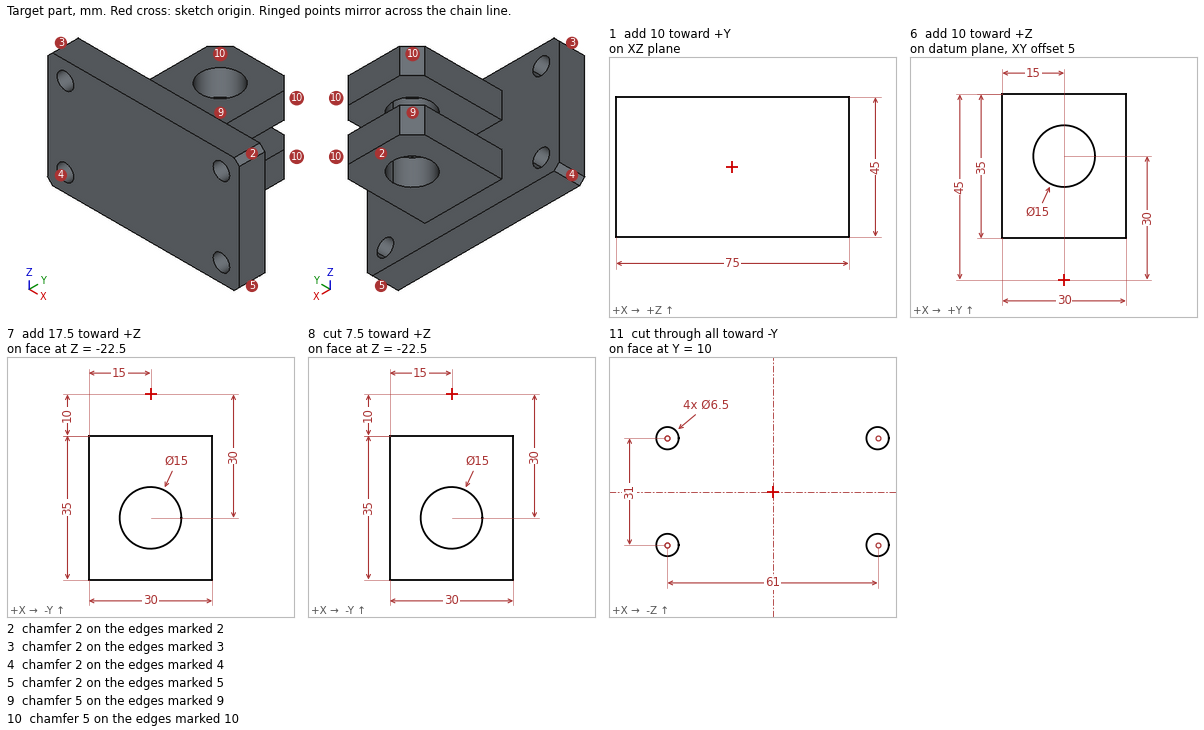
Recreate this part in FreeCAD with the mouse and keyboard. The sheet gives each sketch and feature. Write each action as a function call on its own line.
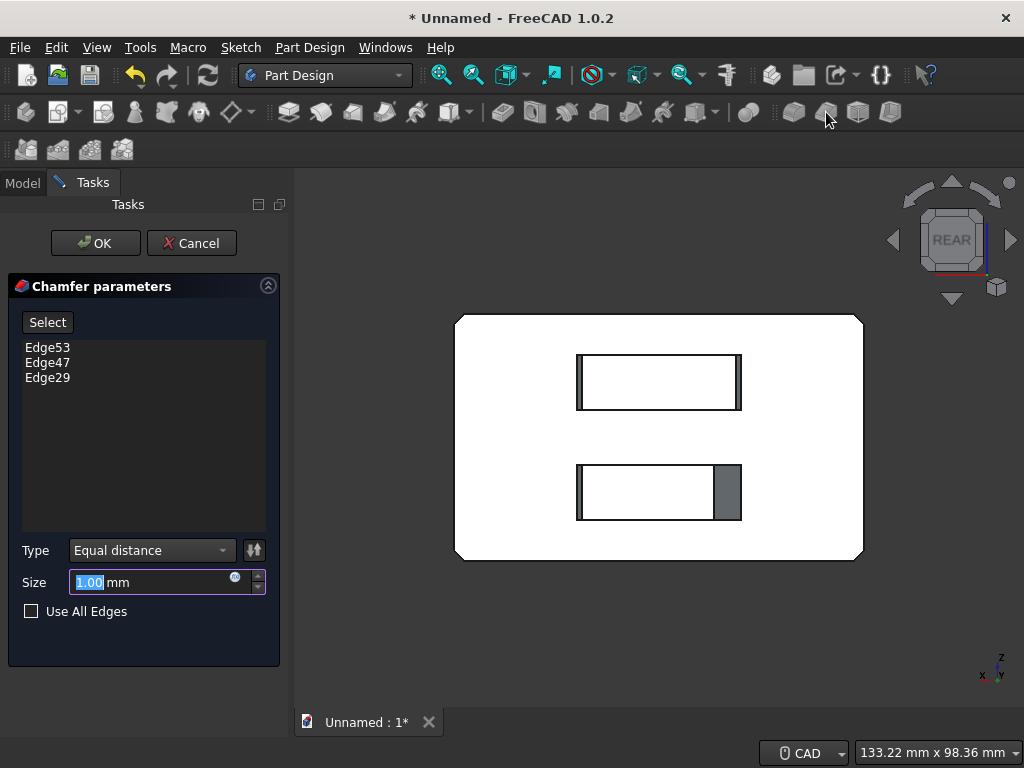
text(5)
key(Tab)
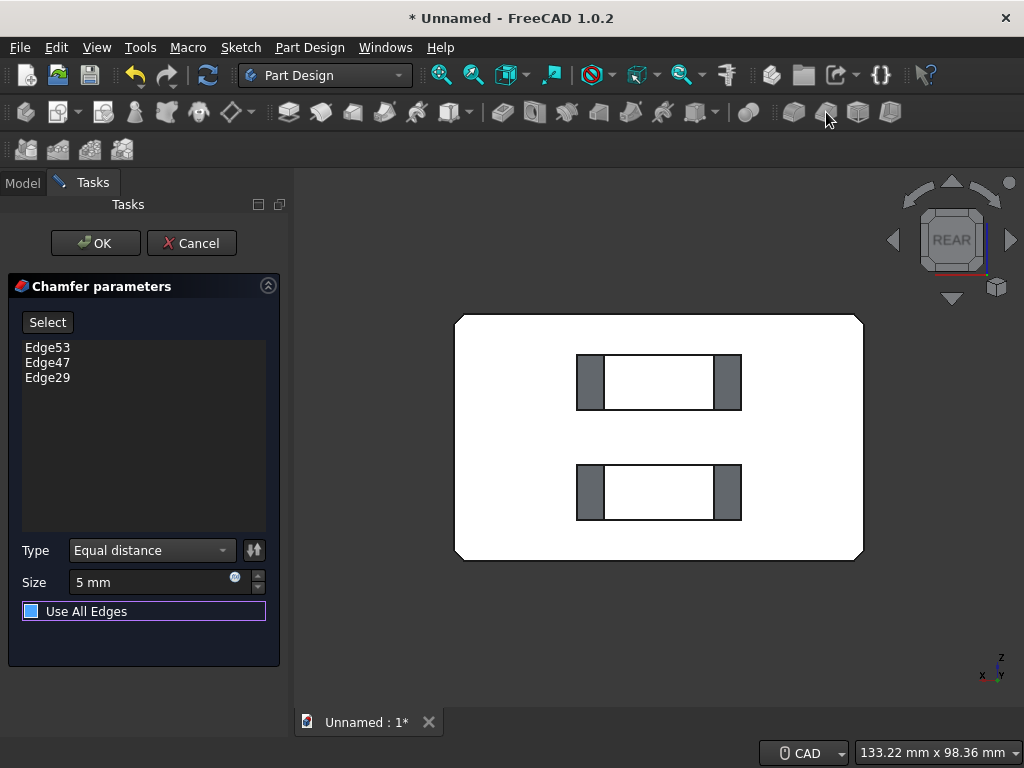
click(96, 243)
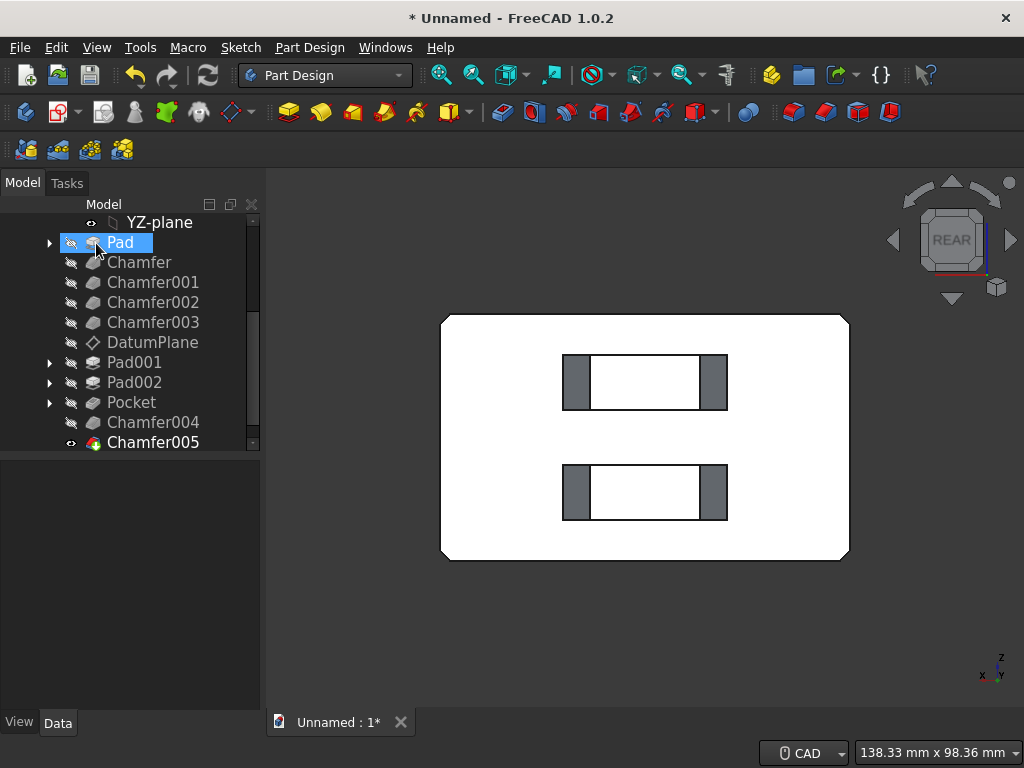
click(762, 436)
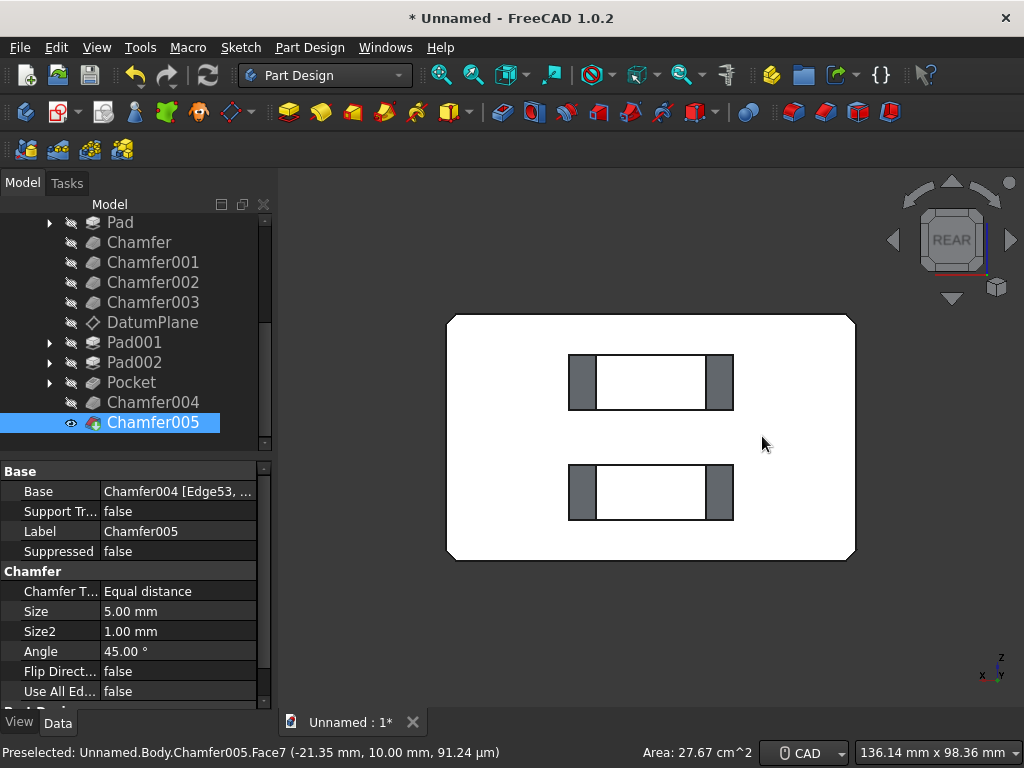
click(58, 112)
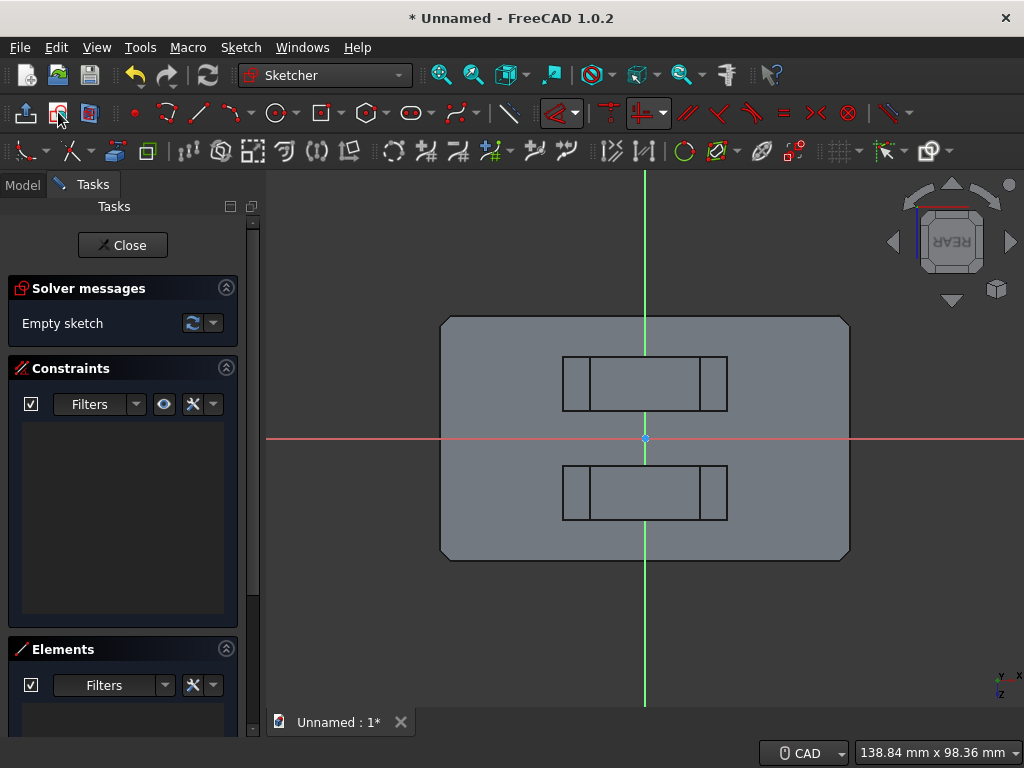
key(g)
key(c)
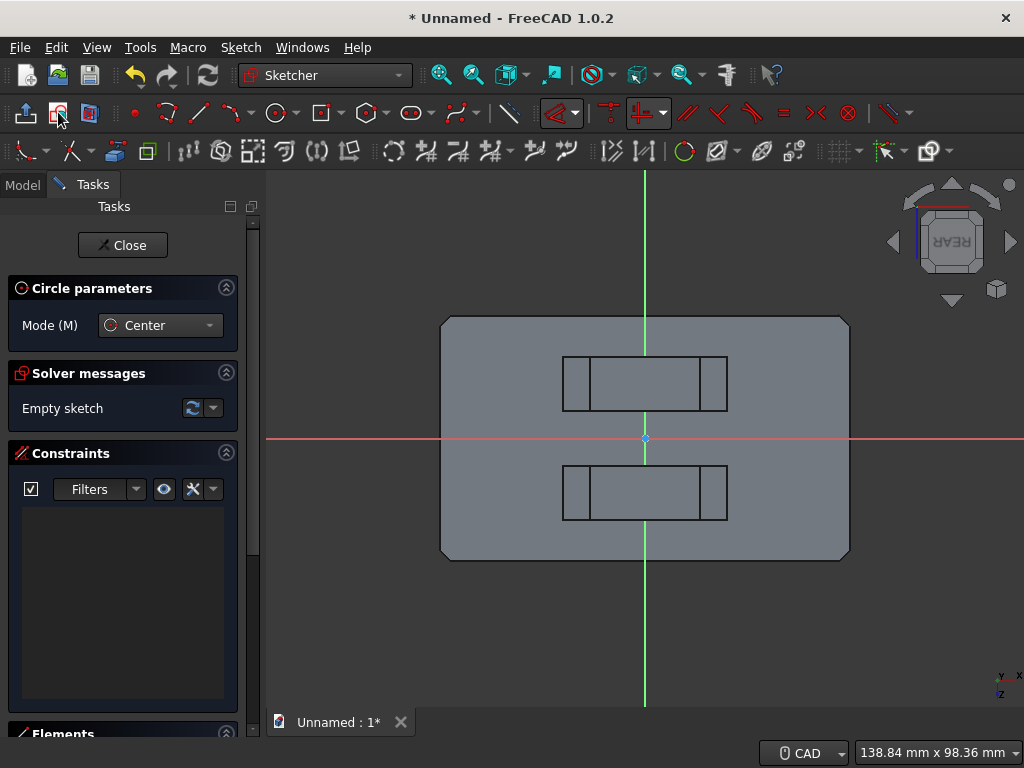
scroll(478, 354, up, 2)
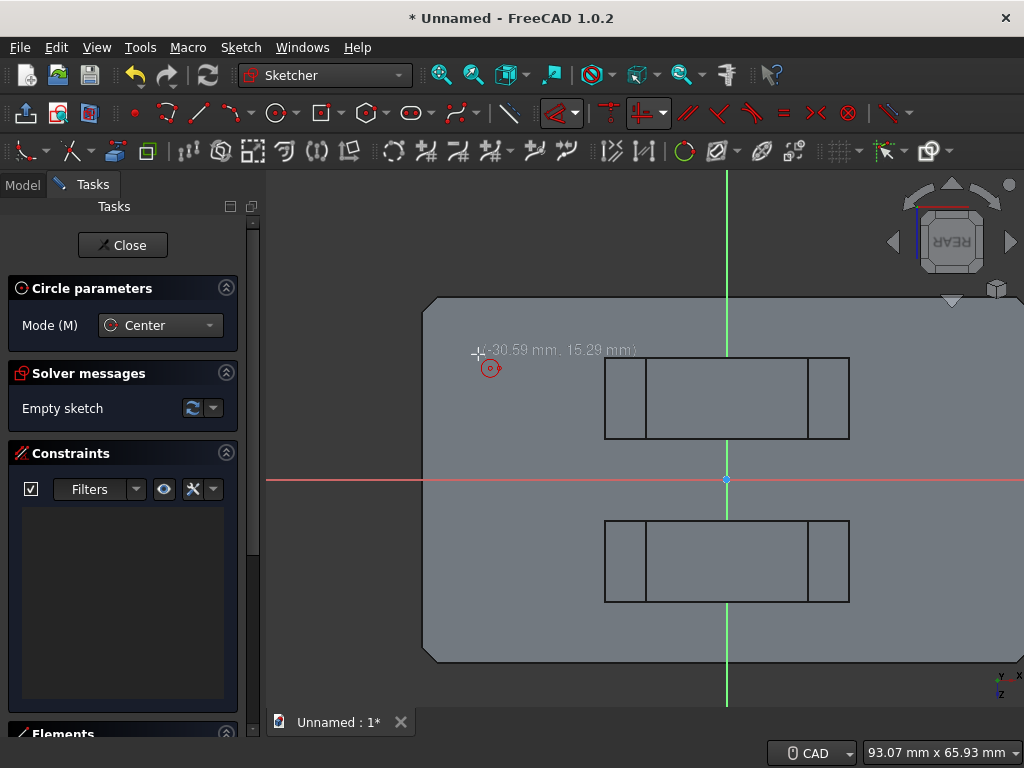
click(479, 354)
click(497, 335)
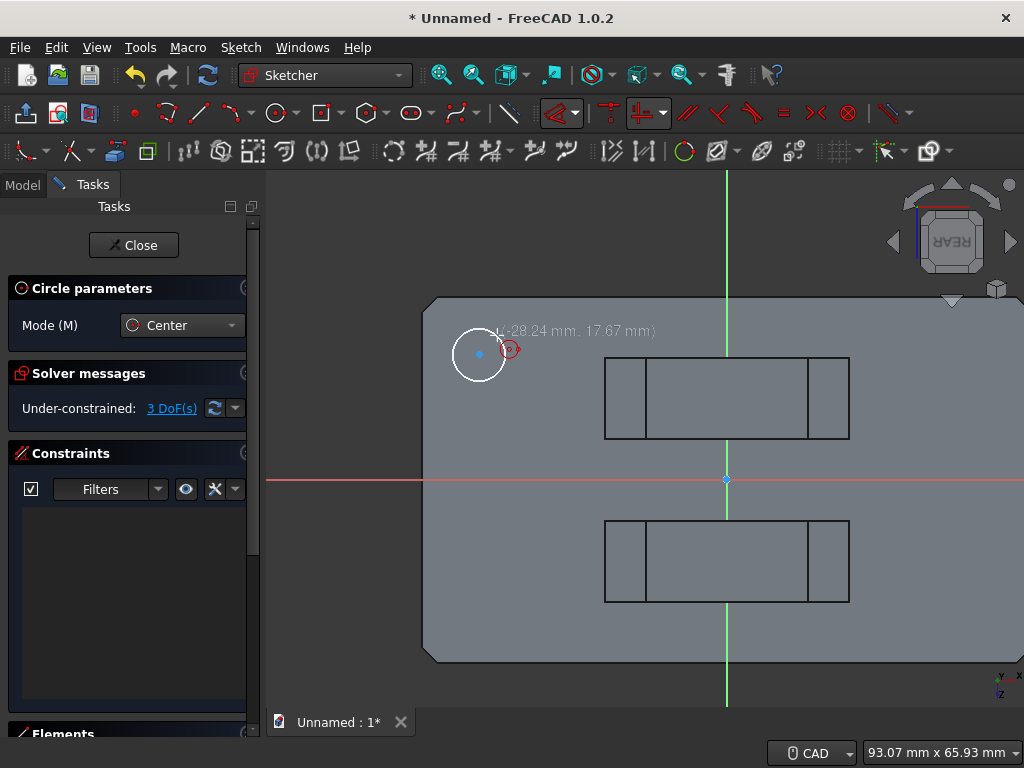
click(479, 606)
click(497, 587)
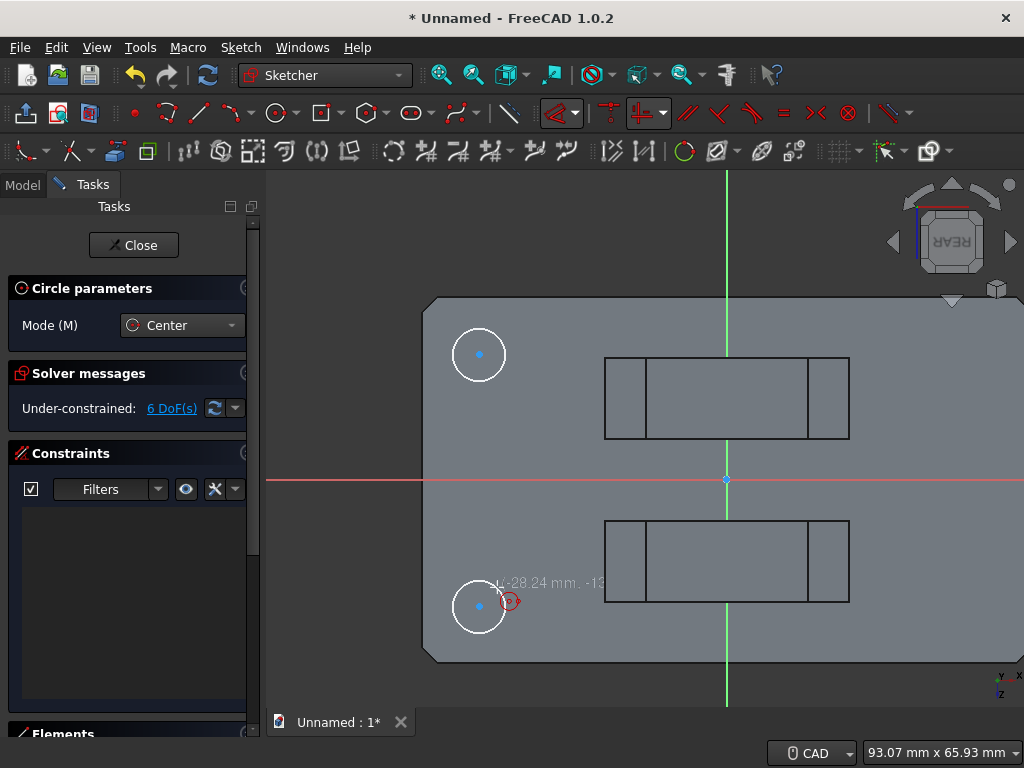
scroll(294, 354, down, 2)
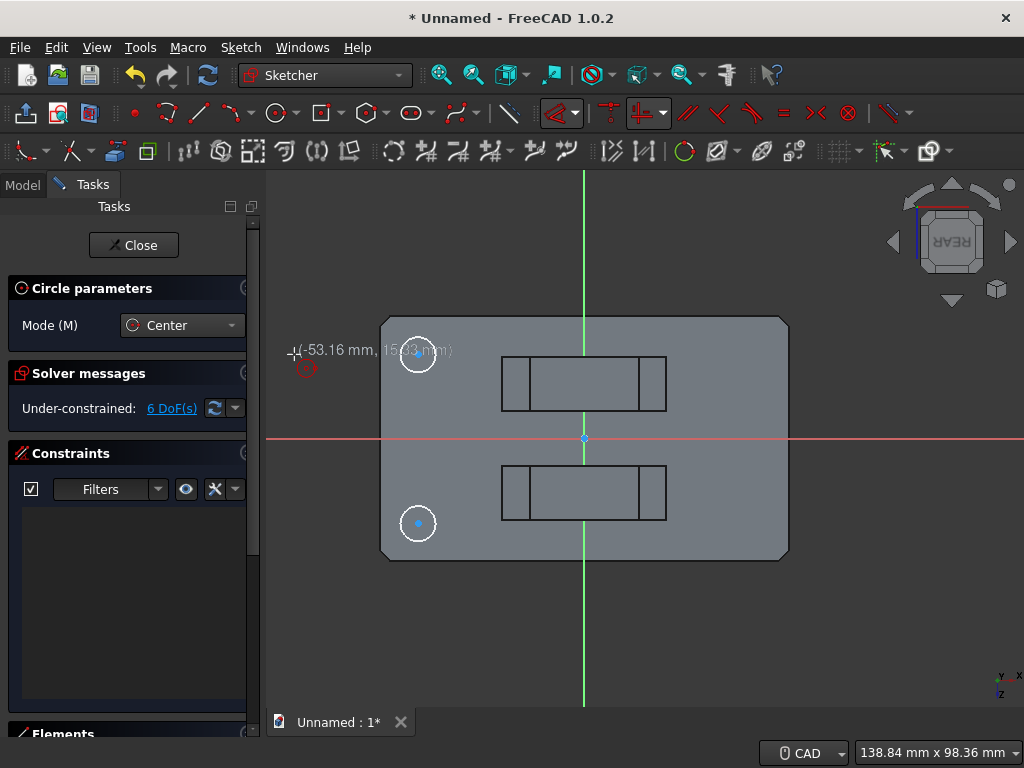
scroll(751, 523, up, 2)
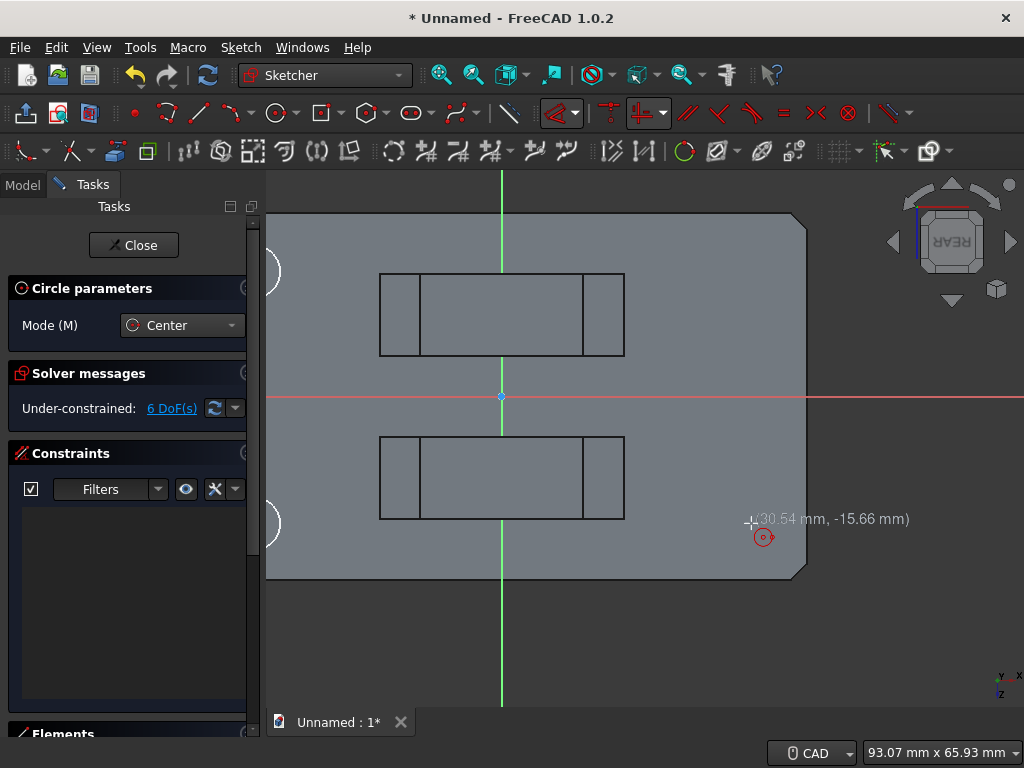
click(750, 523)
click(769, 504)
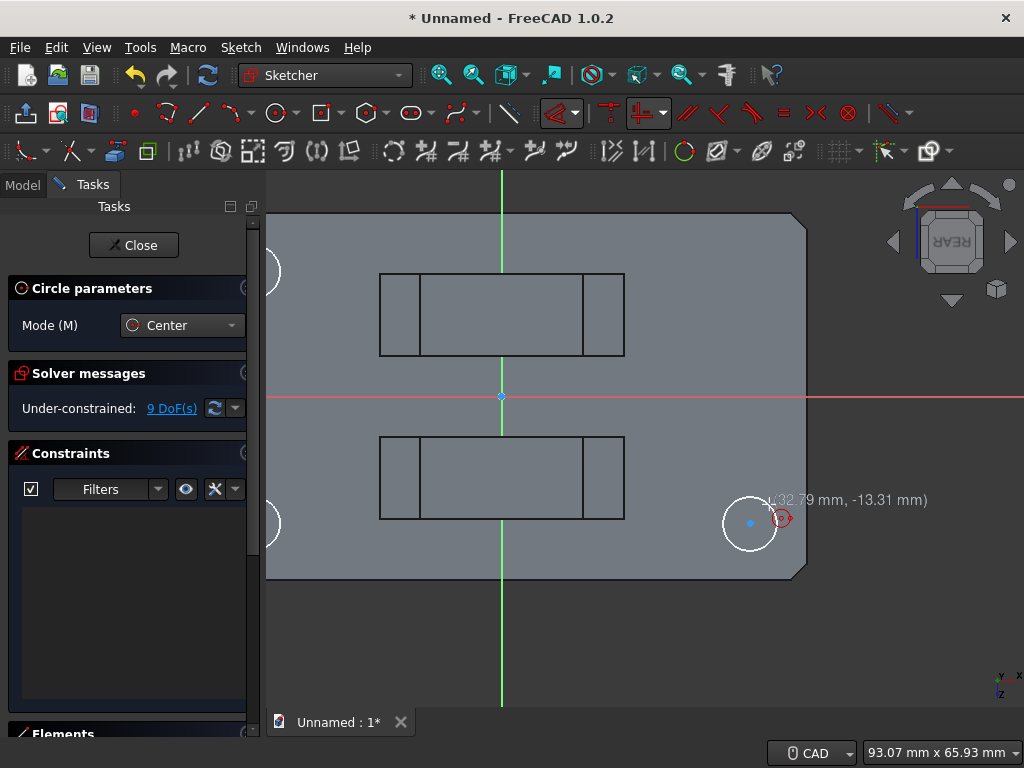
click(750, 270)
click(769, 252)
key(Escape)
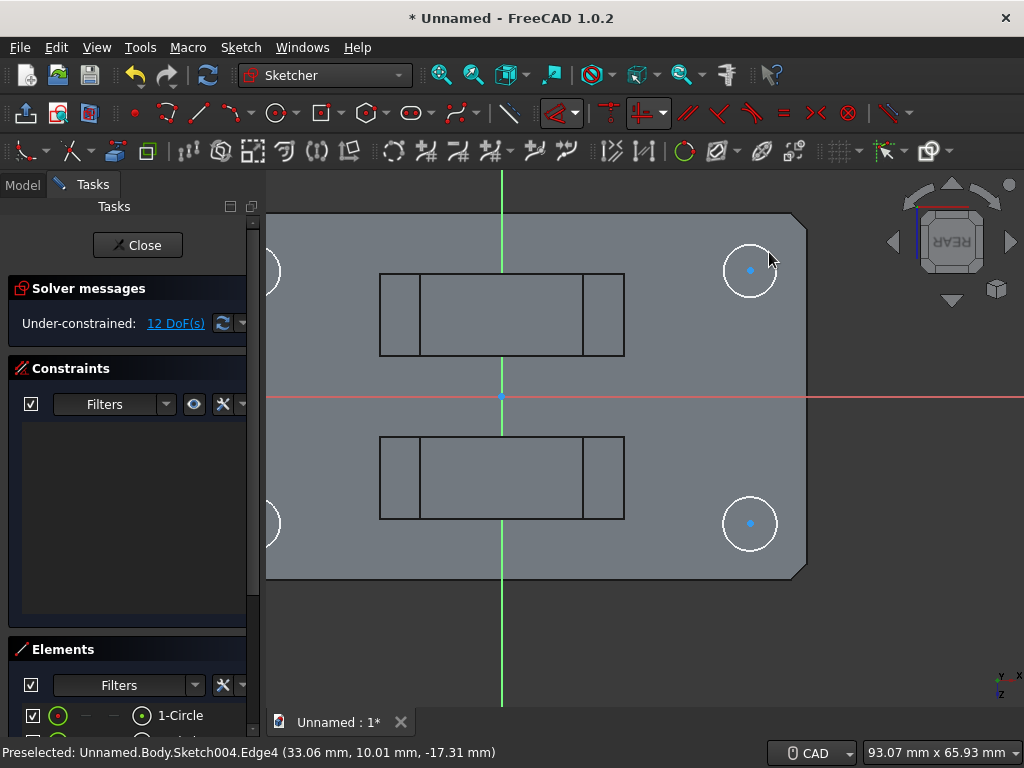
scroll(728, 524, down, 2)